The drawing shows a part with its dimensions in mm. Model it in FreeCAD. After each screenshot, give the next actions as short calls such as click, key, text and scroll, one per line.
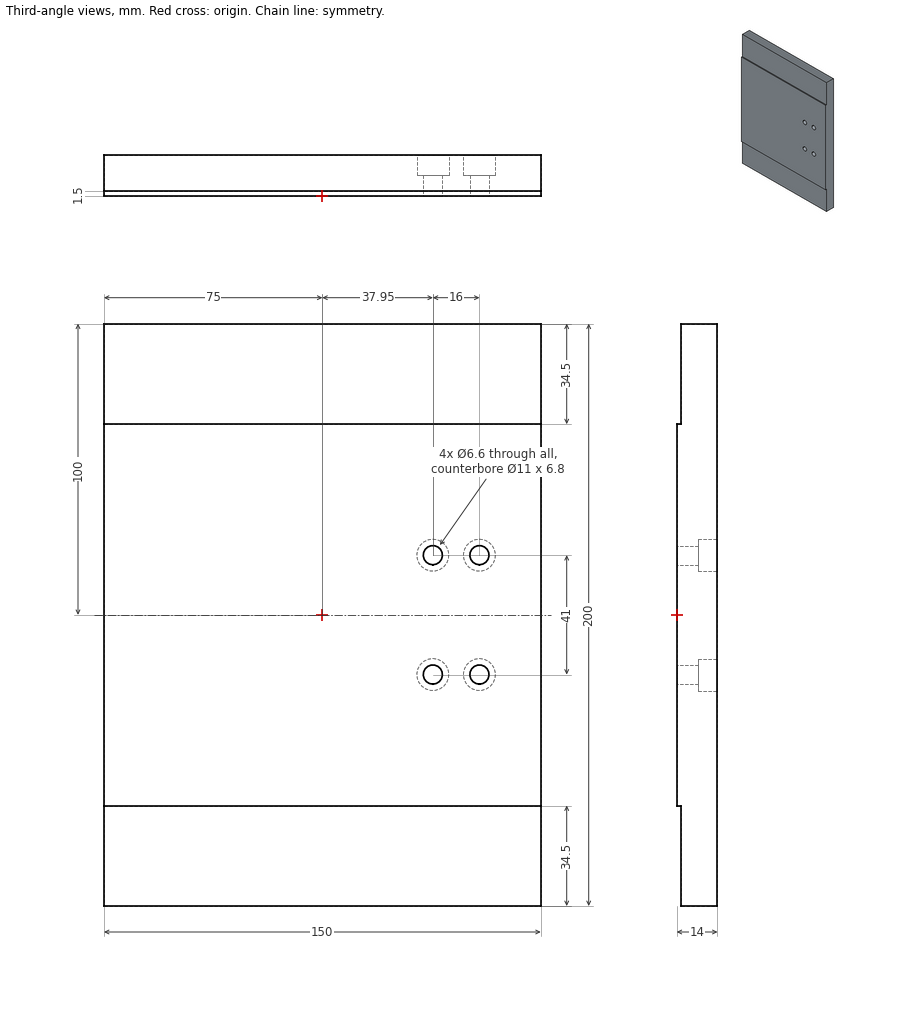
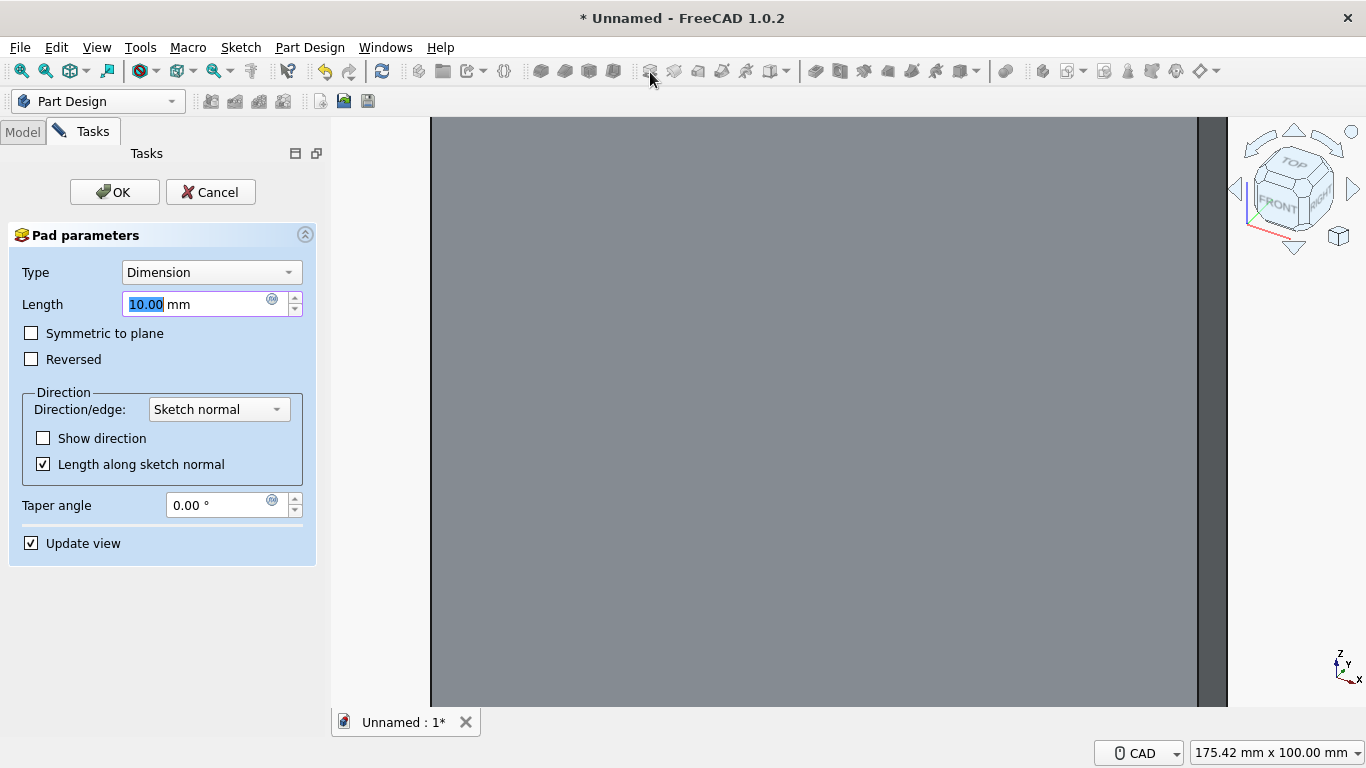
text(14)
key(Tab)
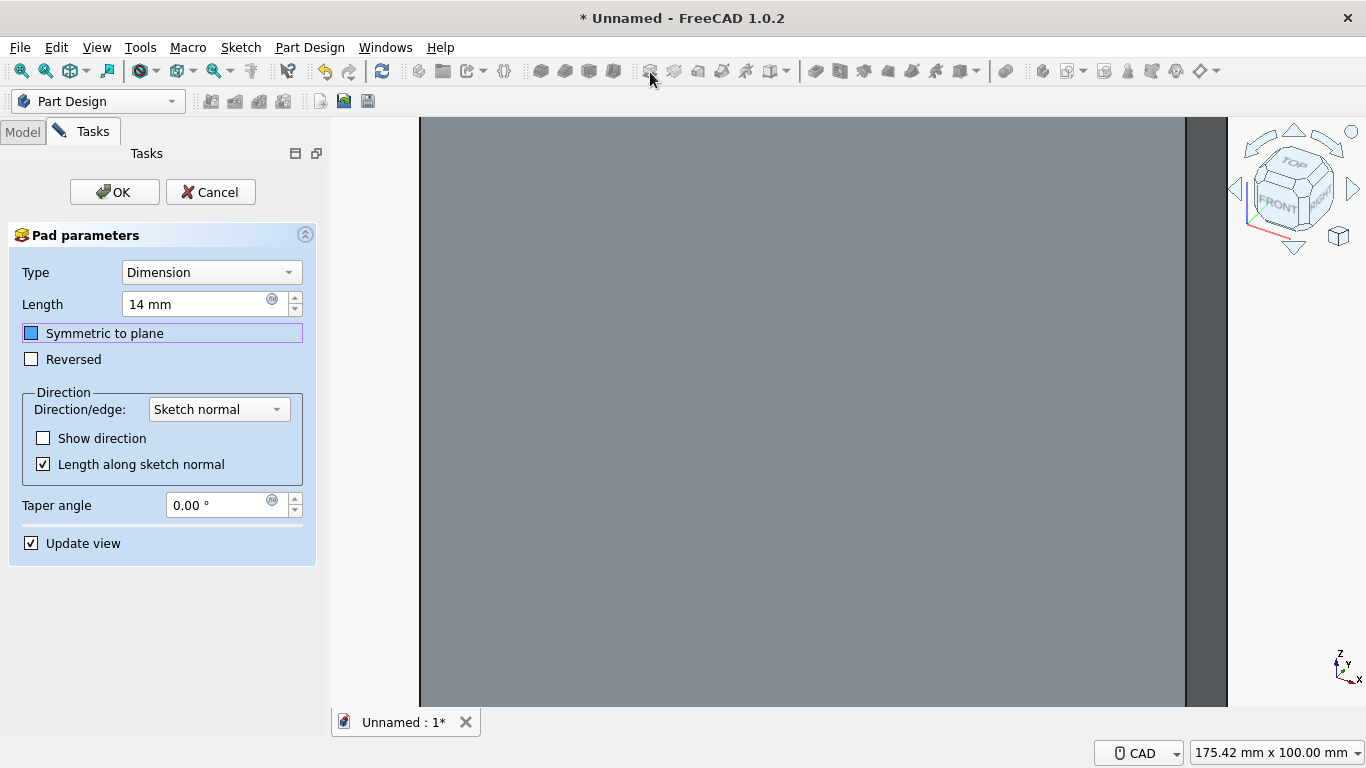
click(30, 359)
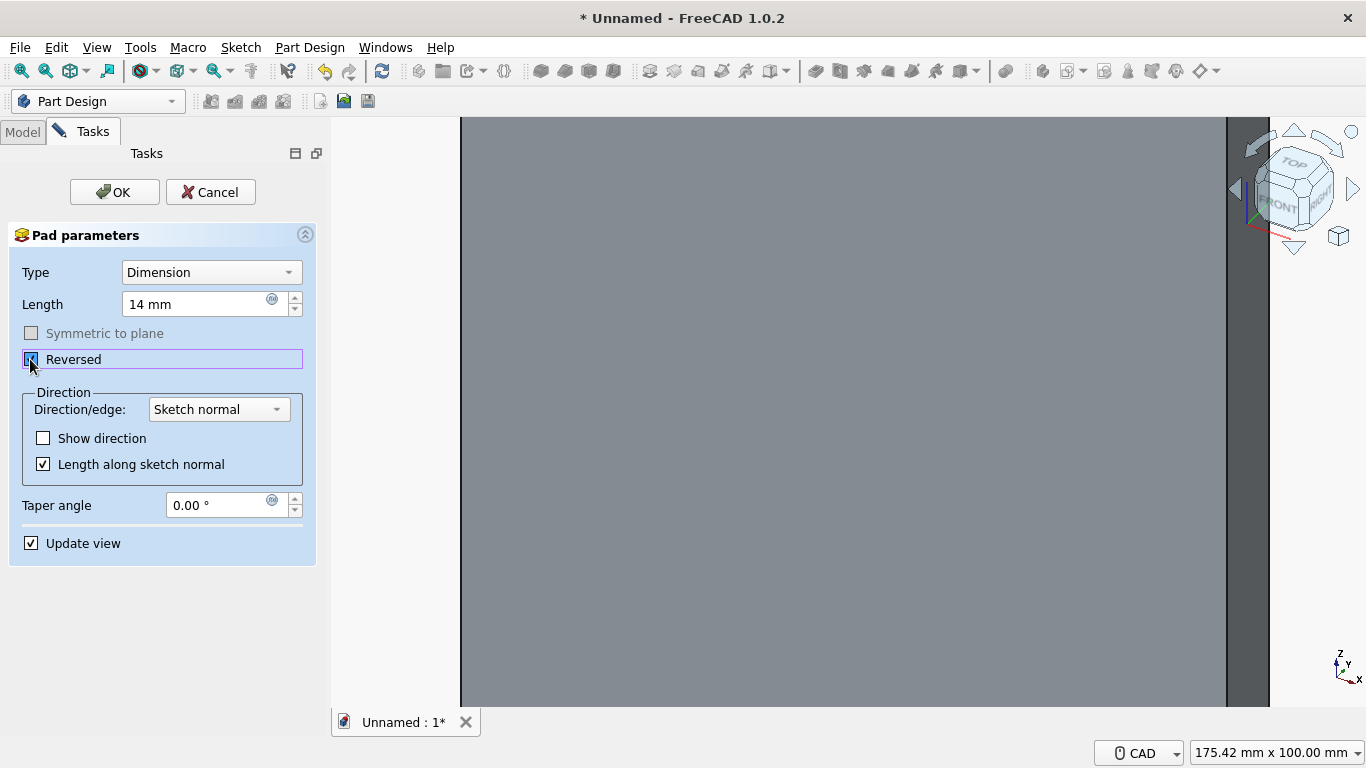
click(115, 192)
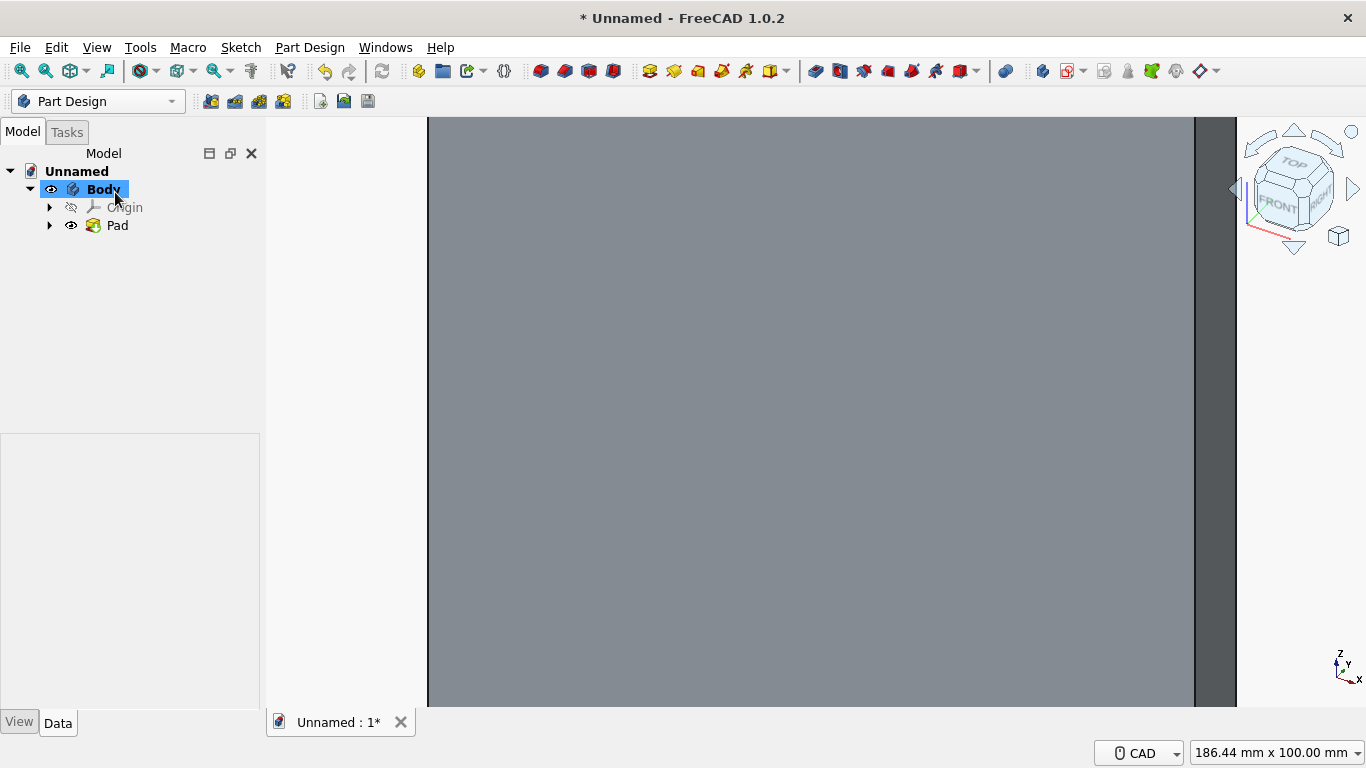
key(v)
key(f)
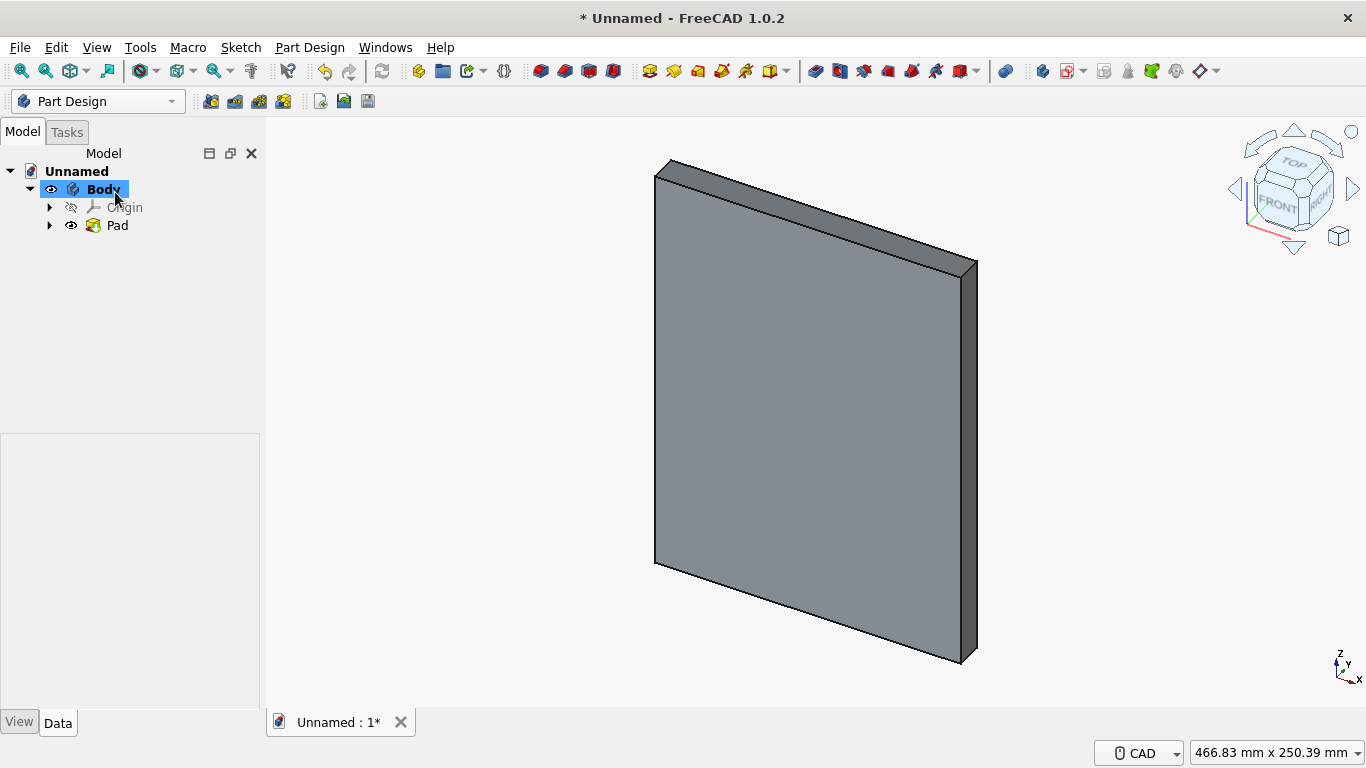
click(808, 419)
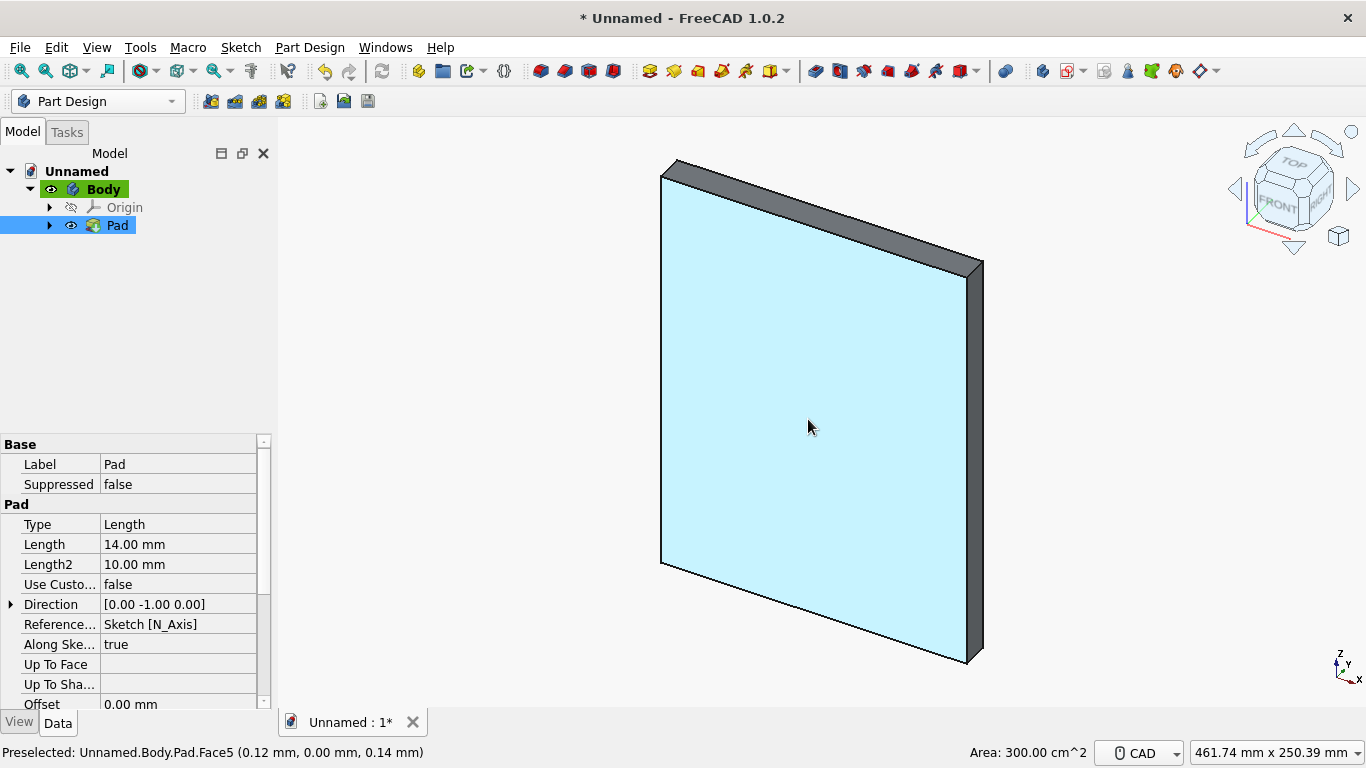
click(1068, 72)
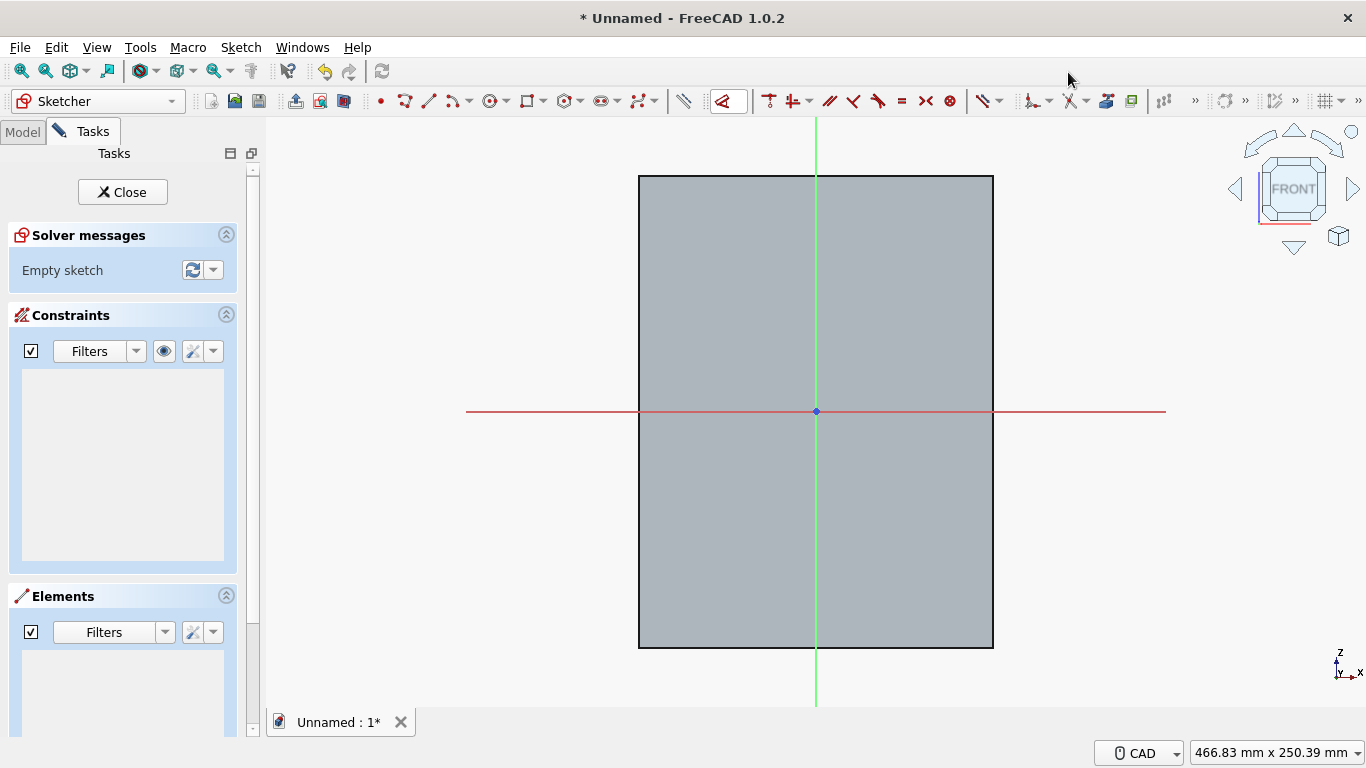
key(g)
key(r)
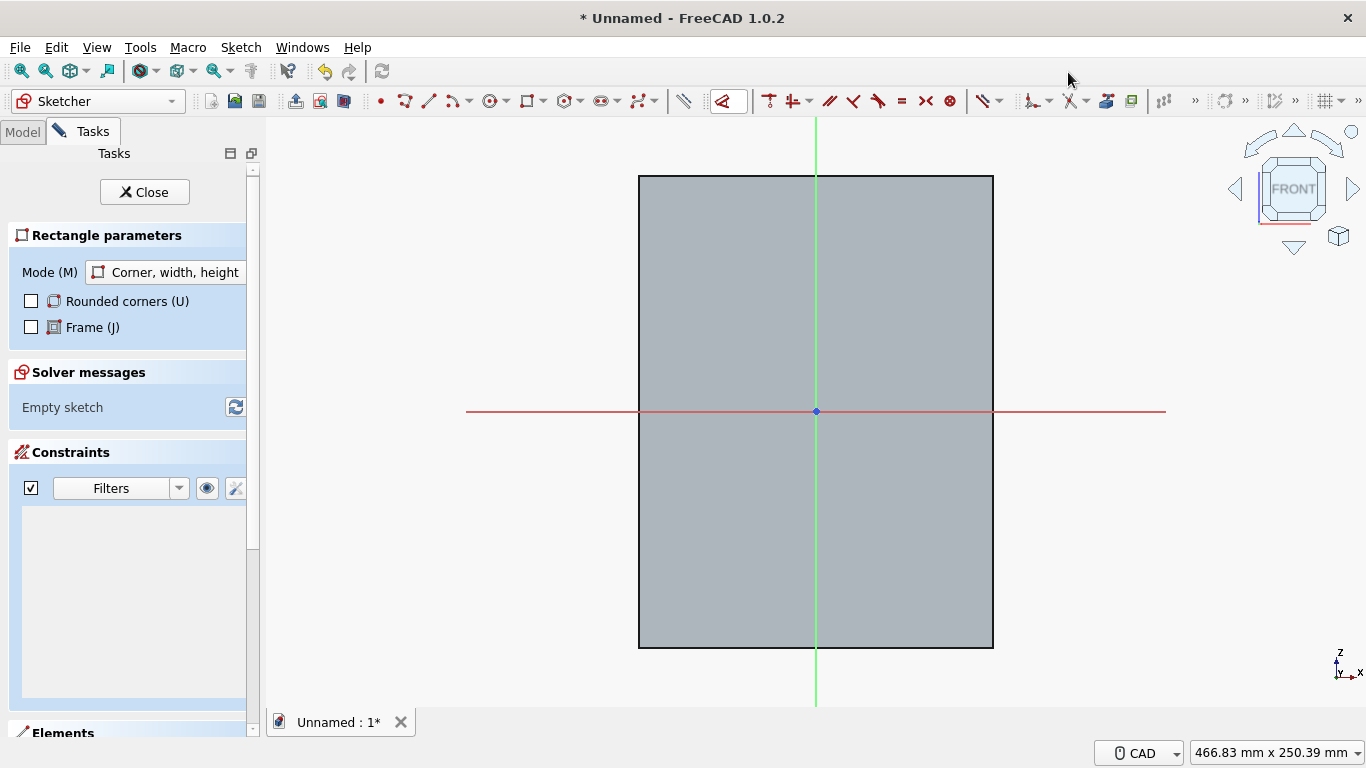
click(639, 176)
move(993, 258)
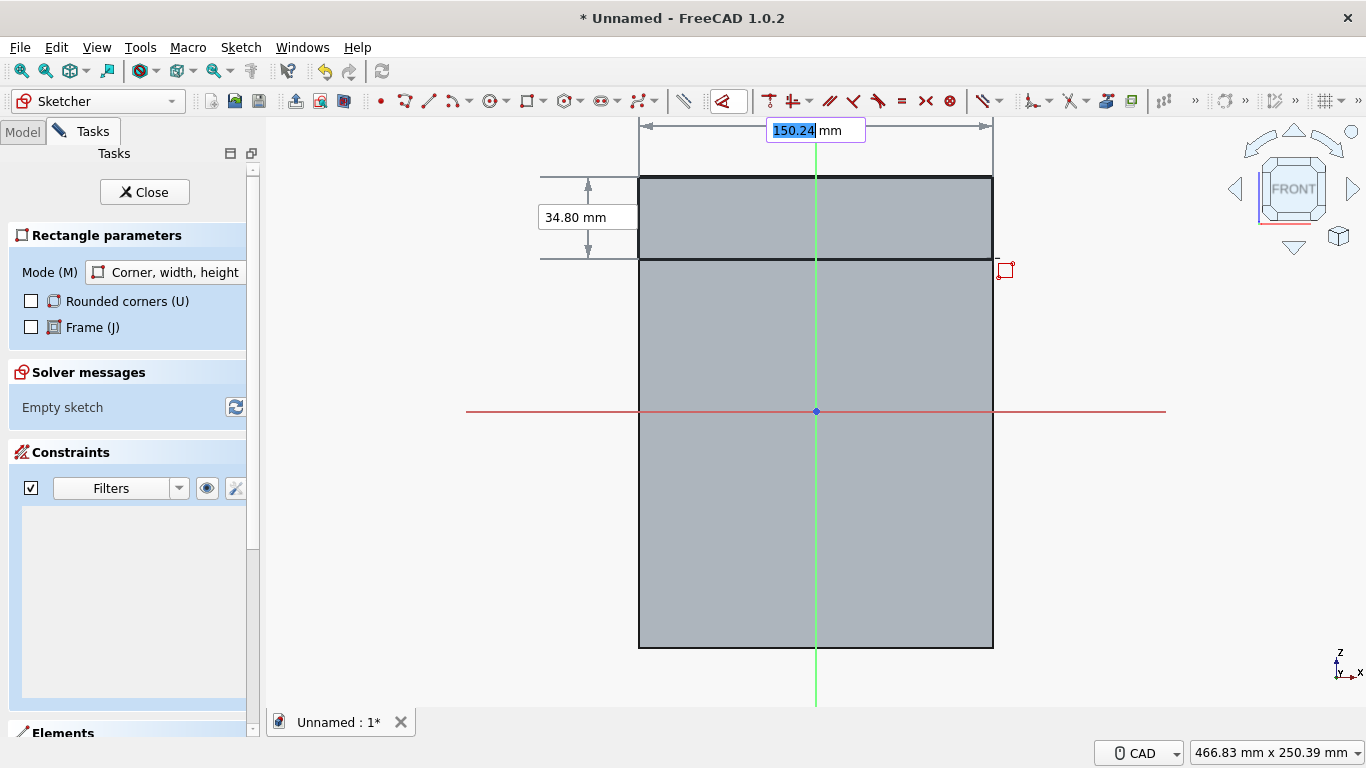
text(150)
key(Tab)
text(34.5)
key(Return)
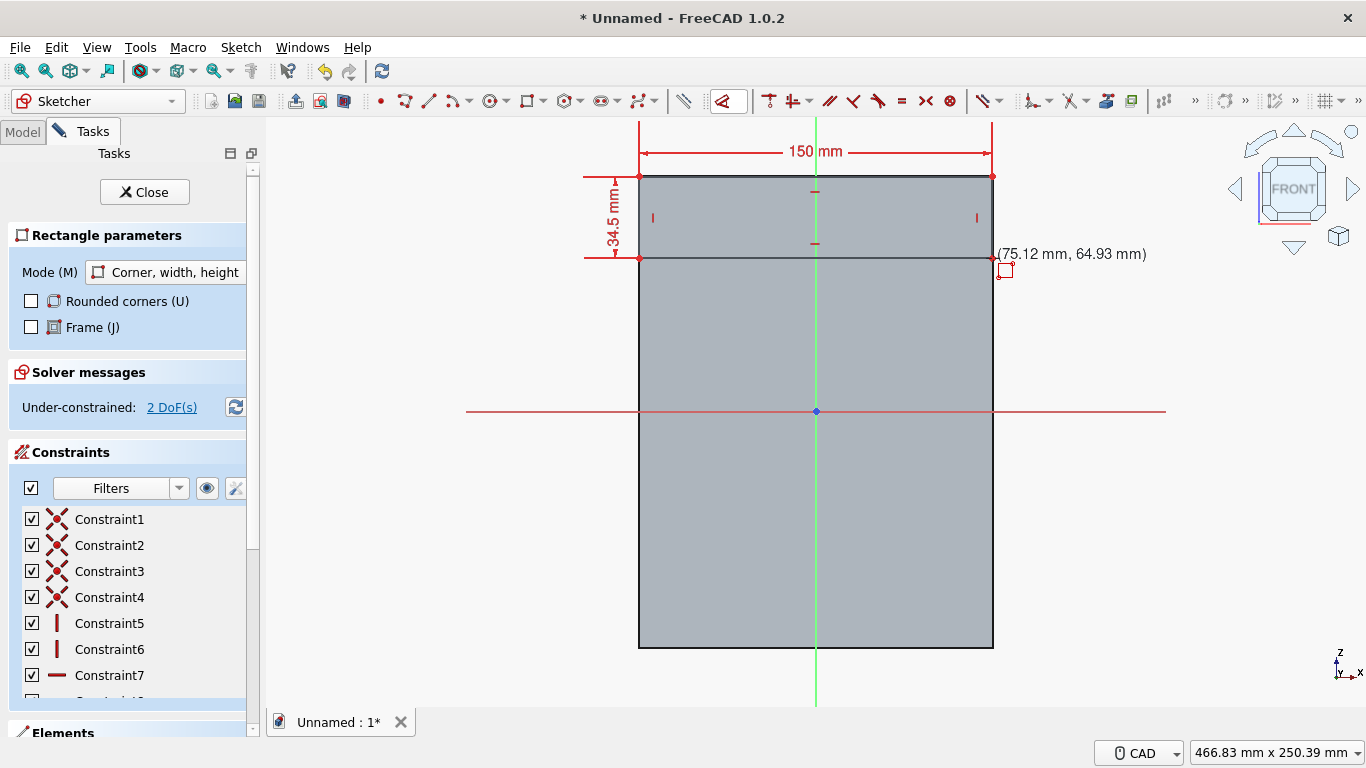
click(639, 566)
move(993, 648)